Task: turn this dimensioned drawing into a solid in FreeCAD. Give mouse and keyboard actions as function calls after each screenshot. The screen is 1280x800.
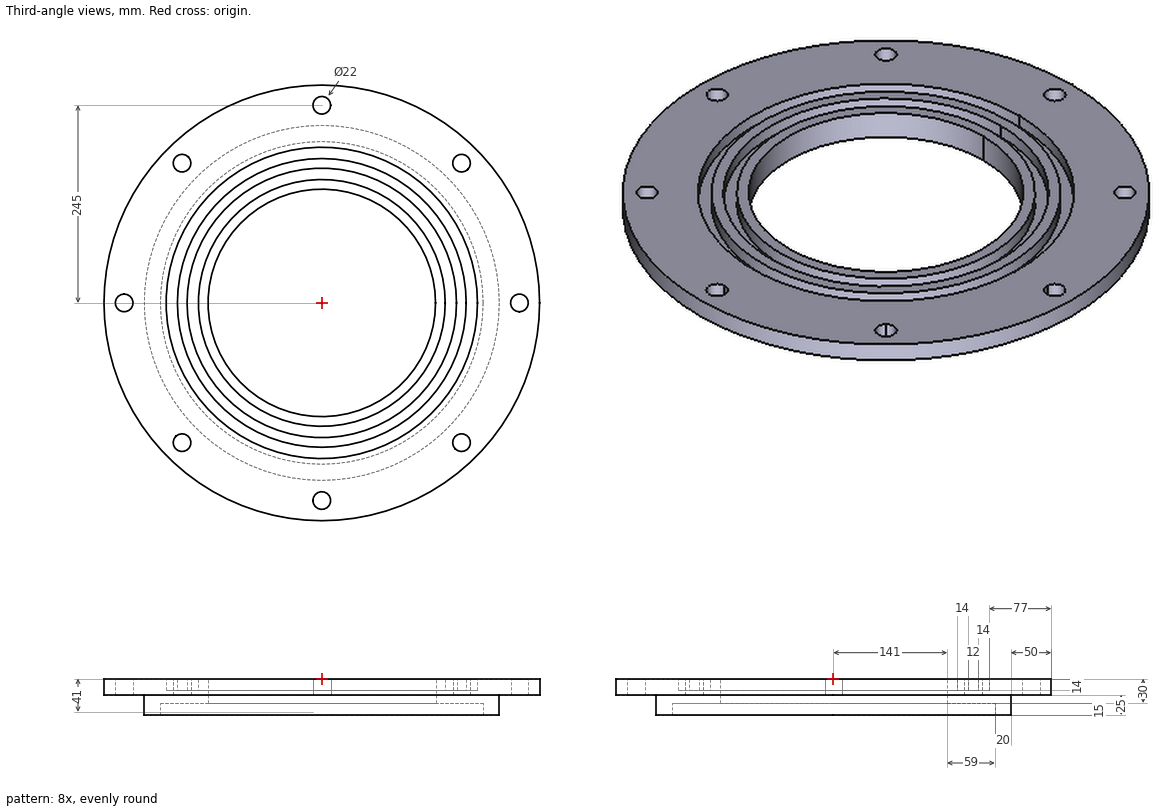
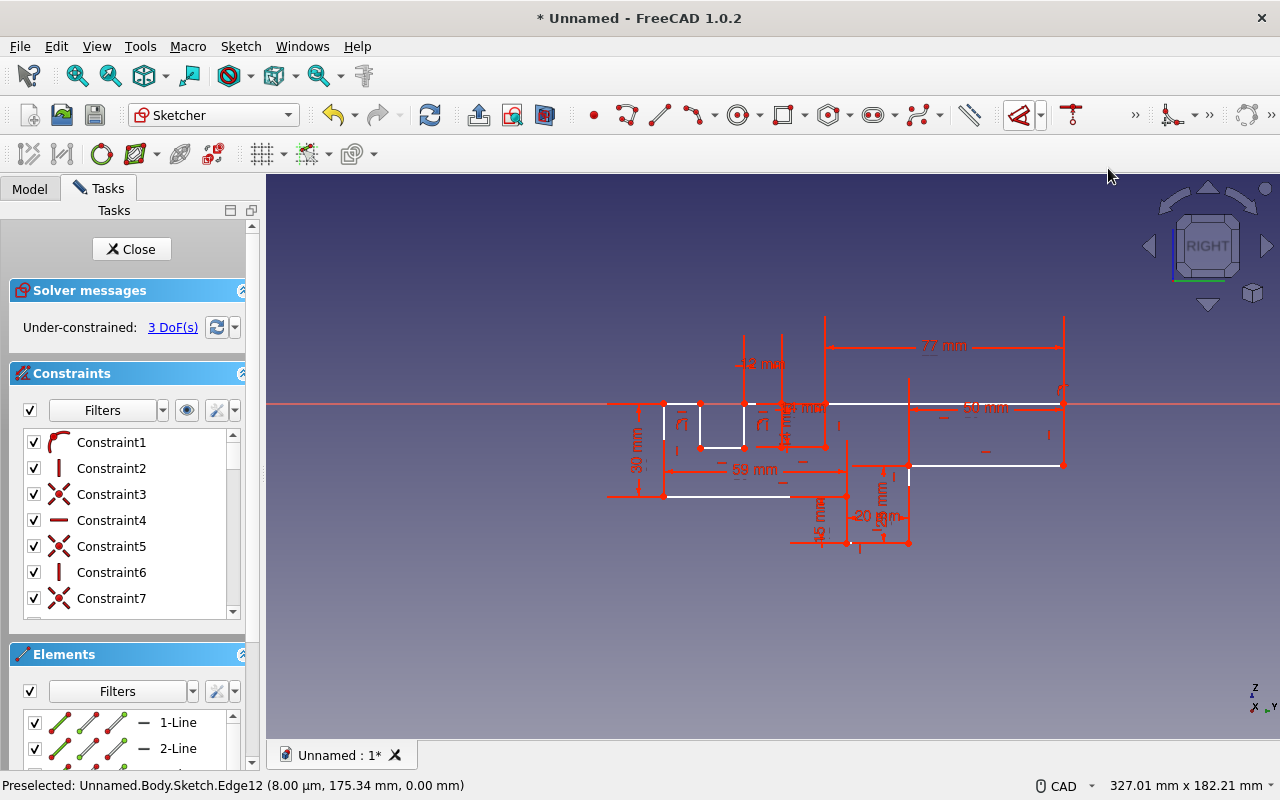
click(744, 417)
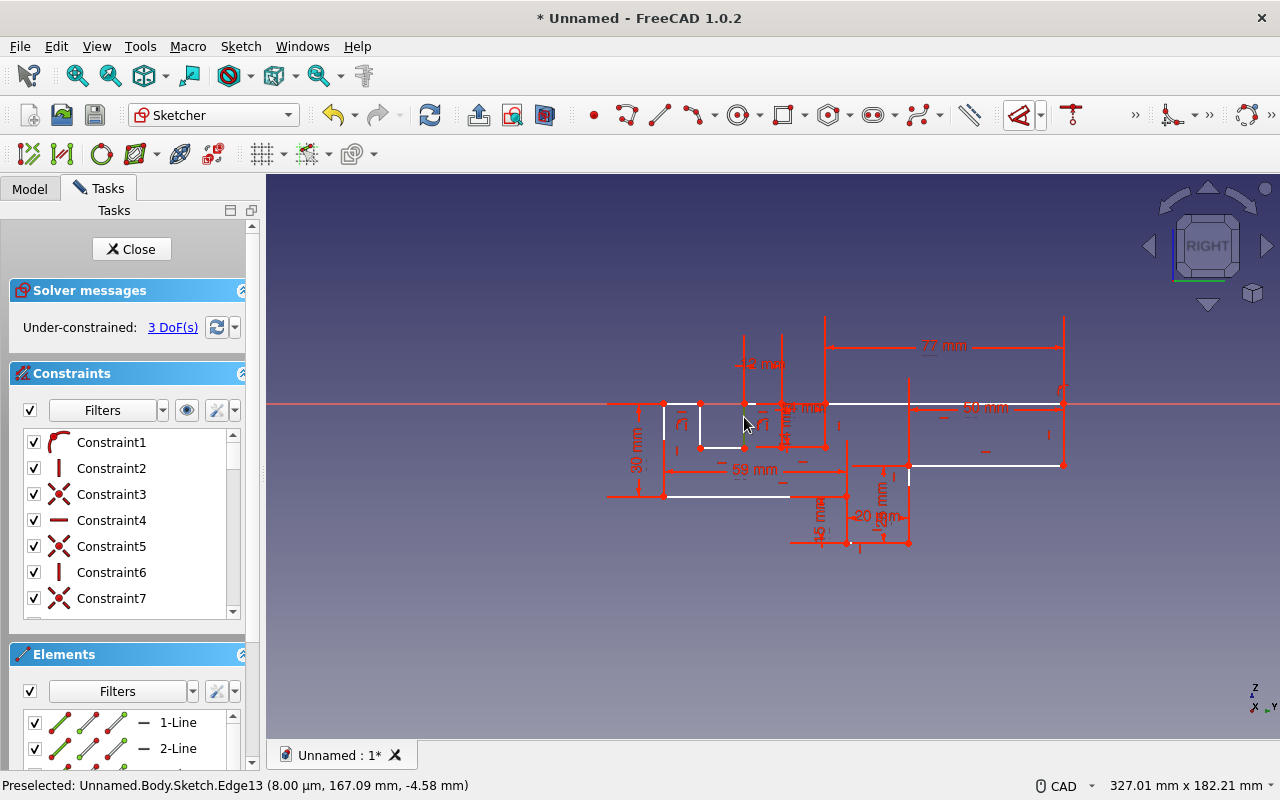
key(i)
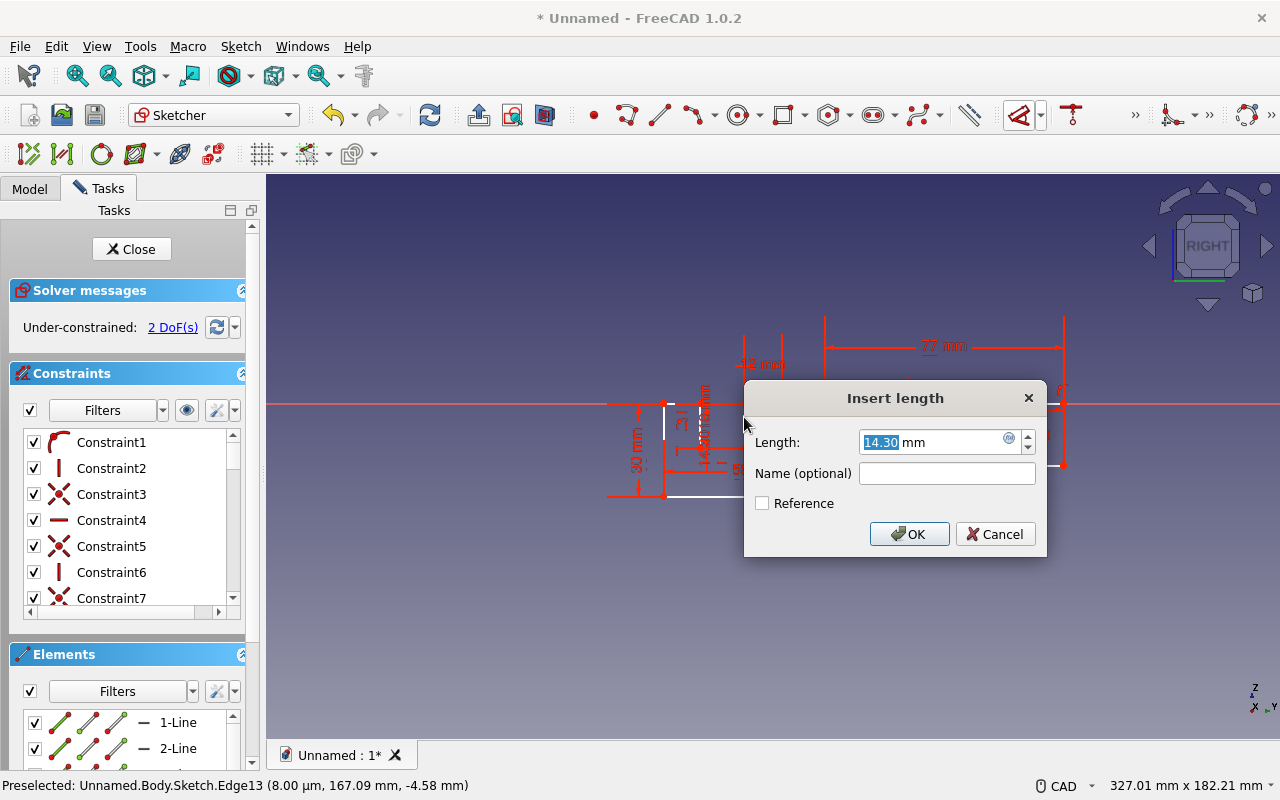
text(14)
key(Return)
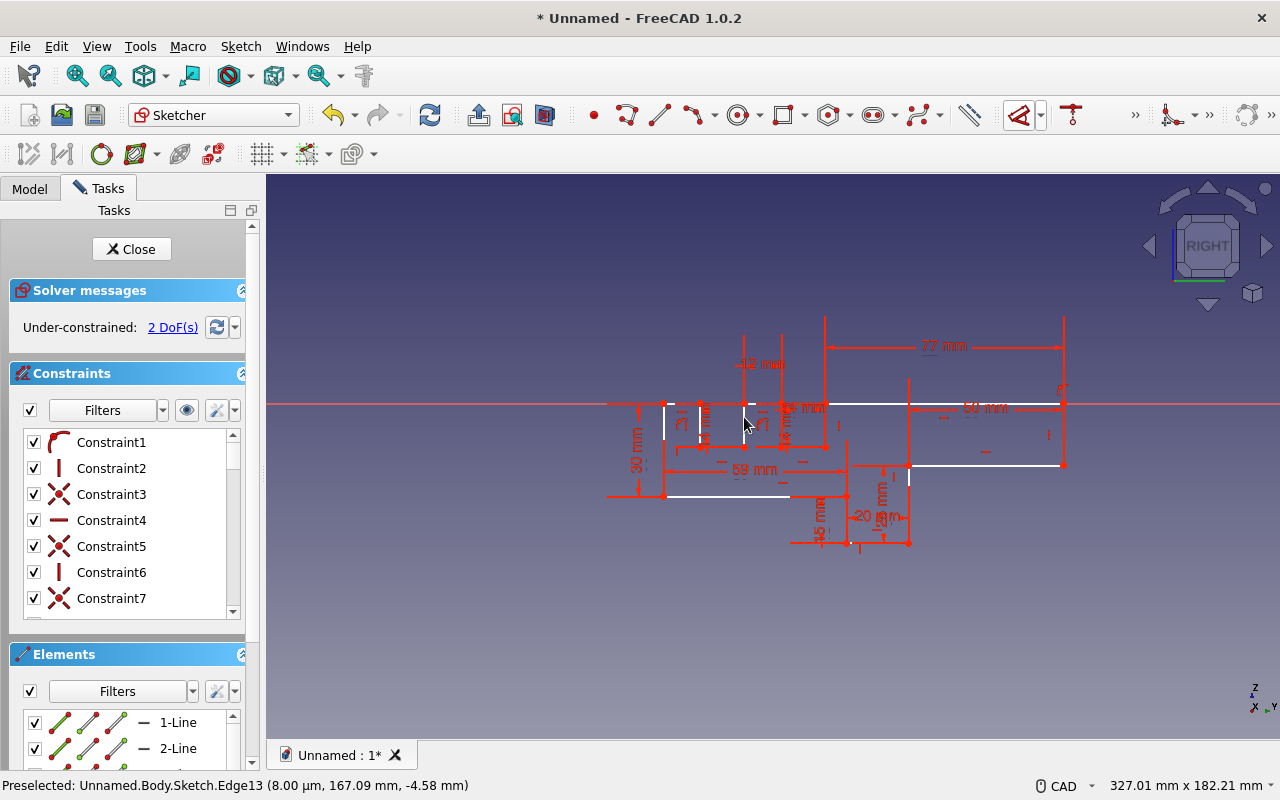
click(731, 447)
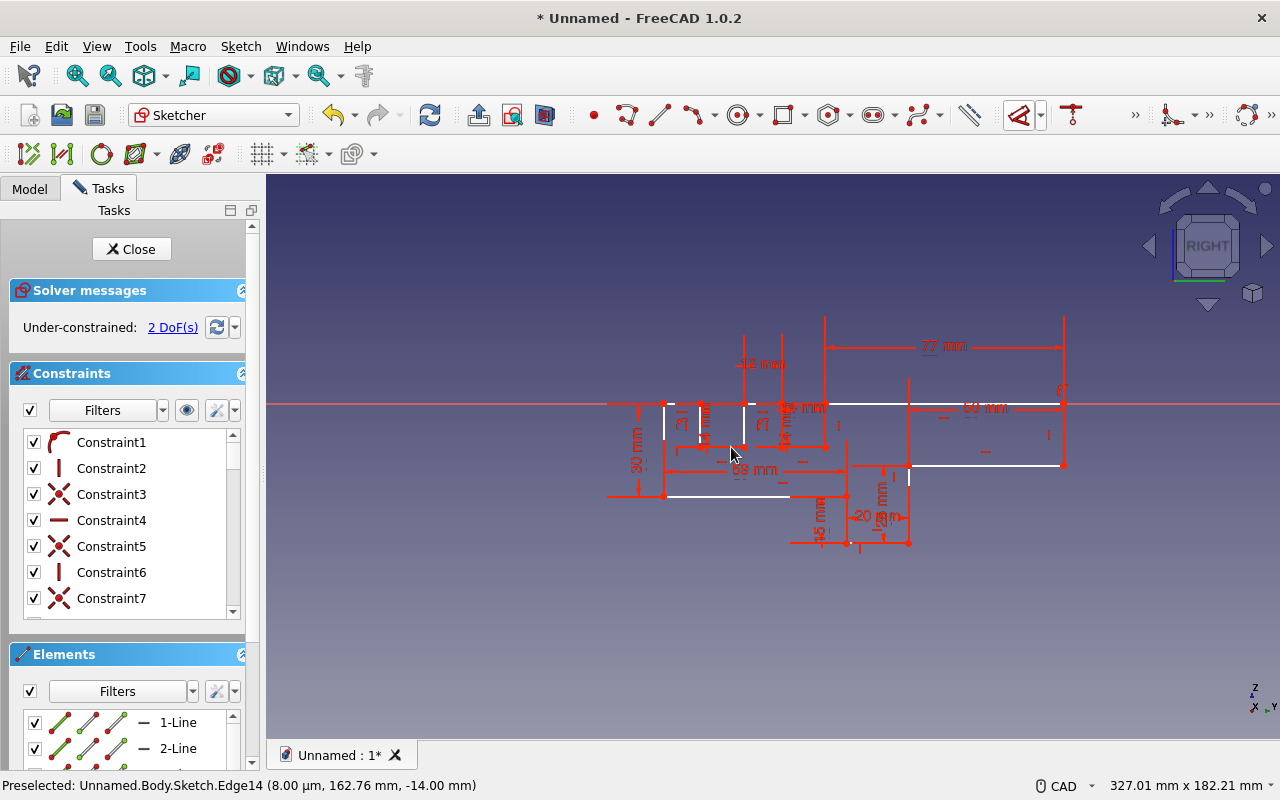
click(1040, 116)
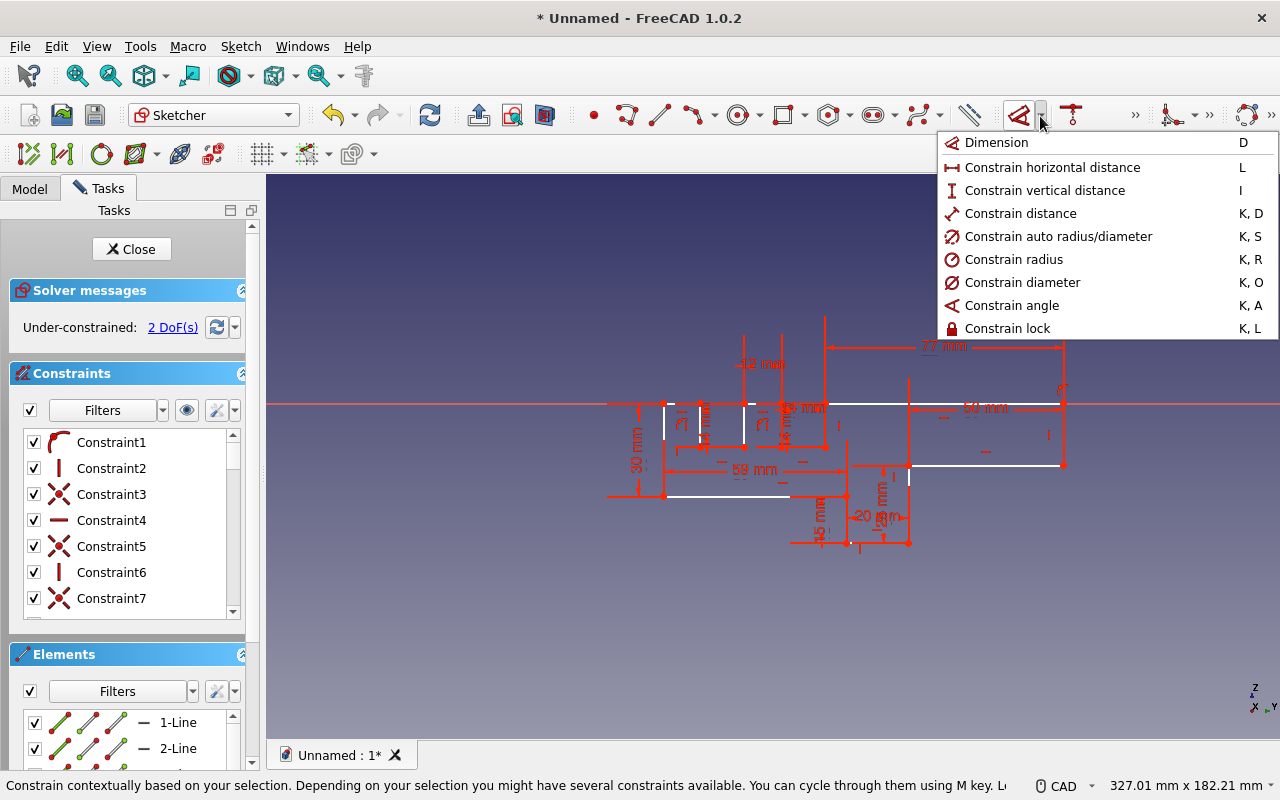
click(1108, 168)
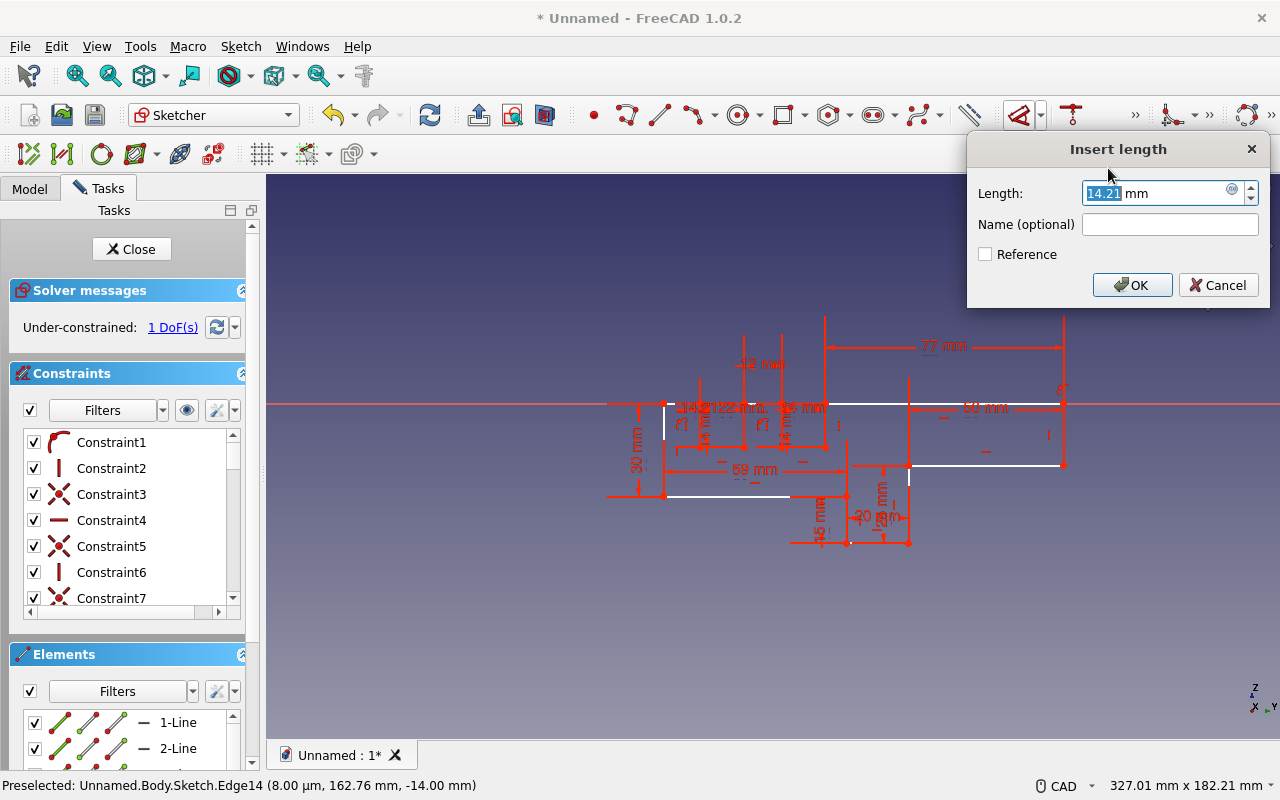
text(14)
key(Return)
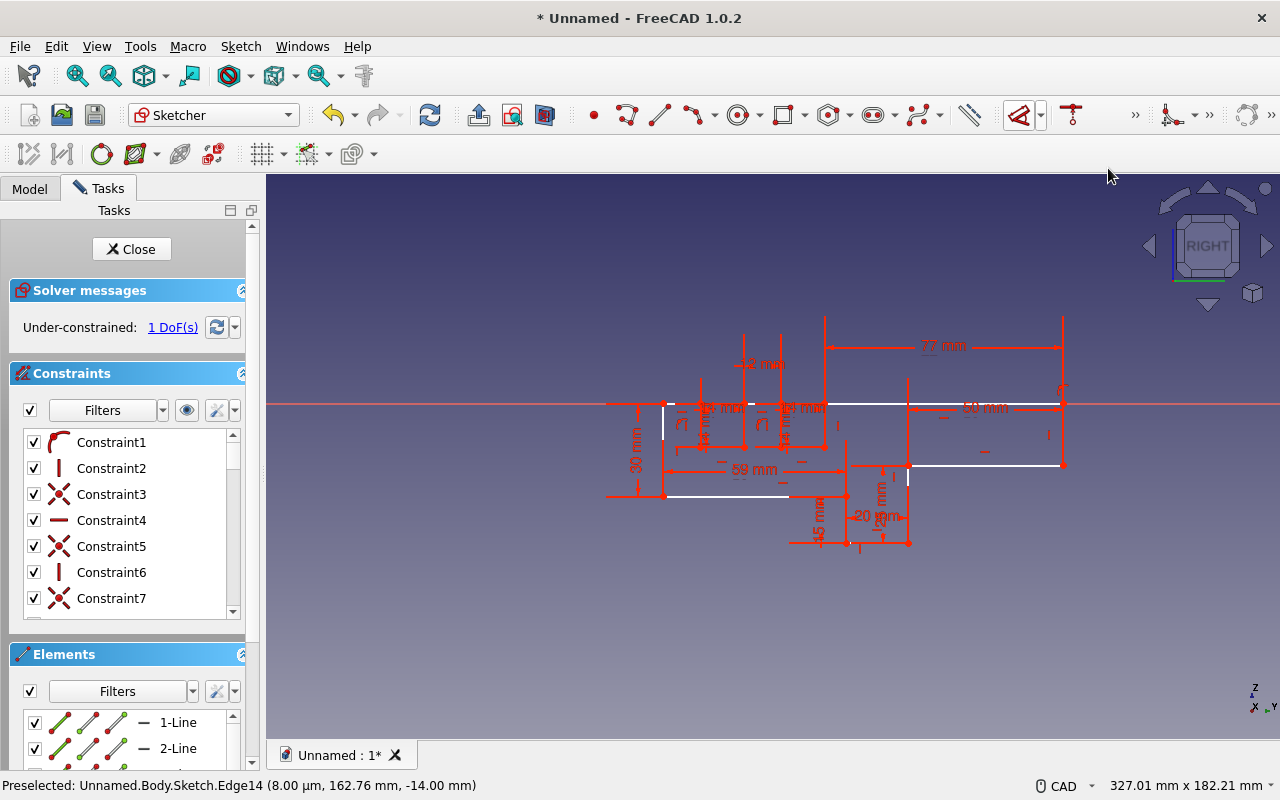
click(663, 404)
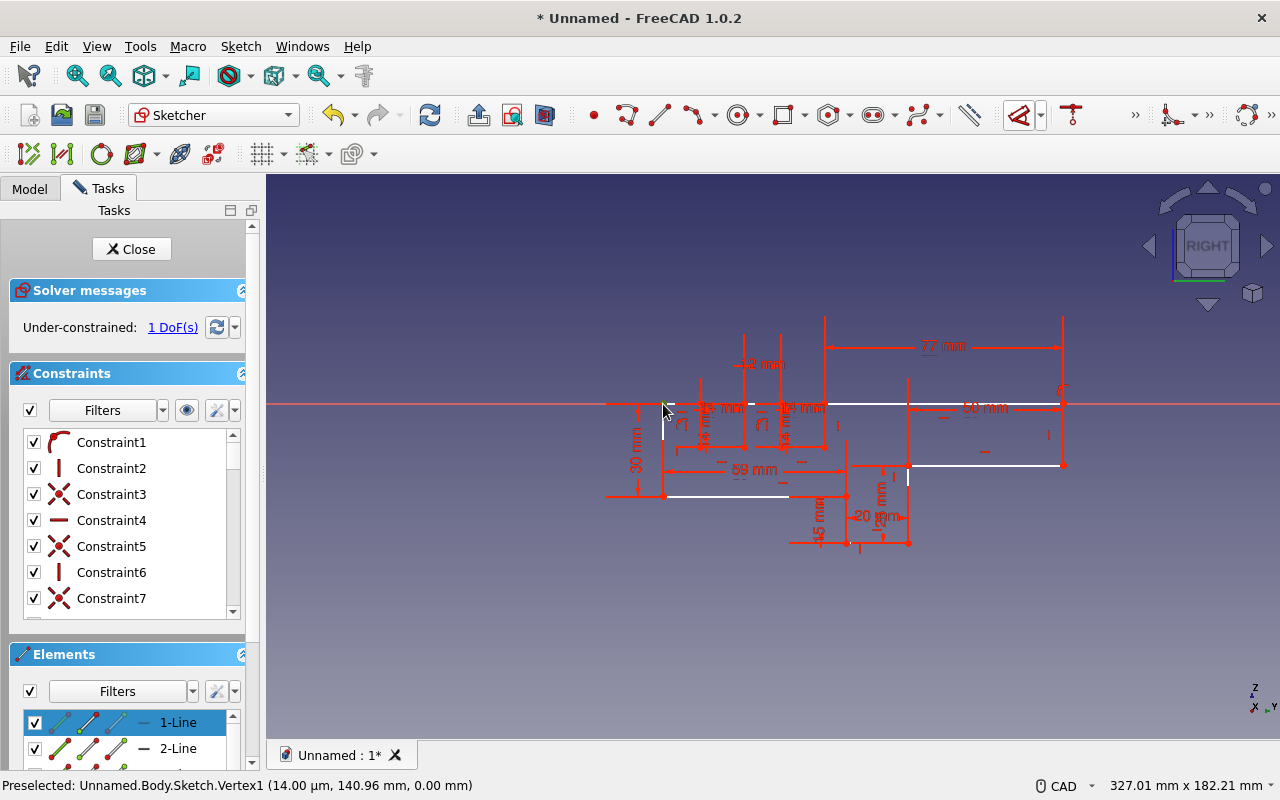
click(1040, 116)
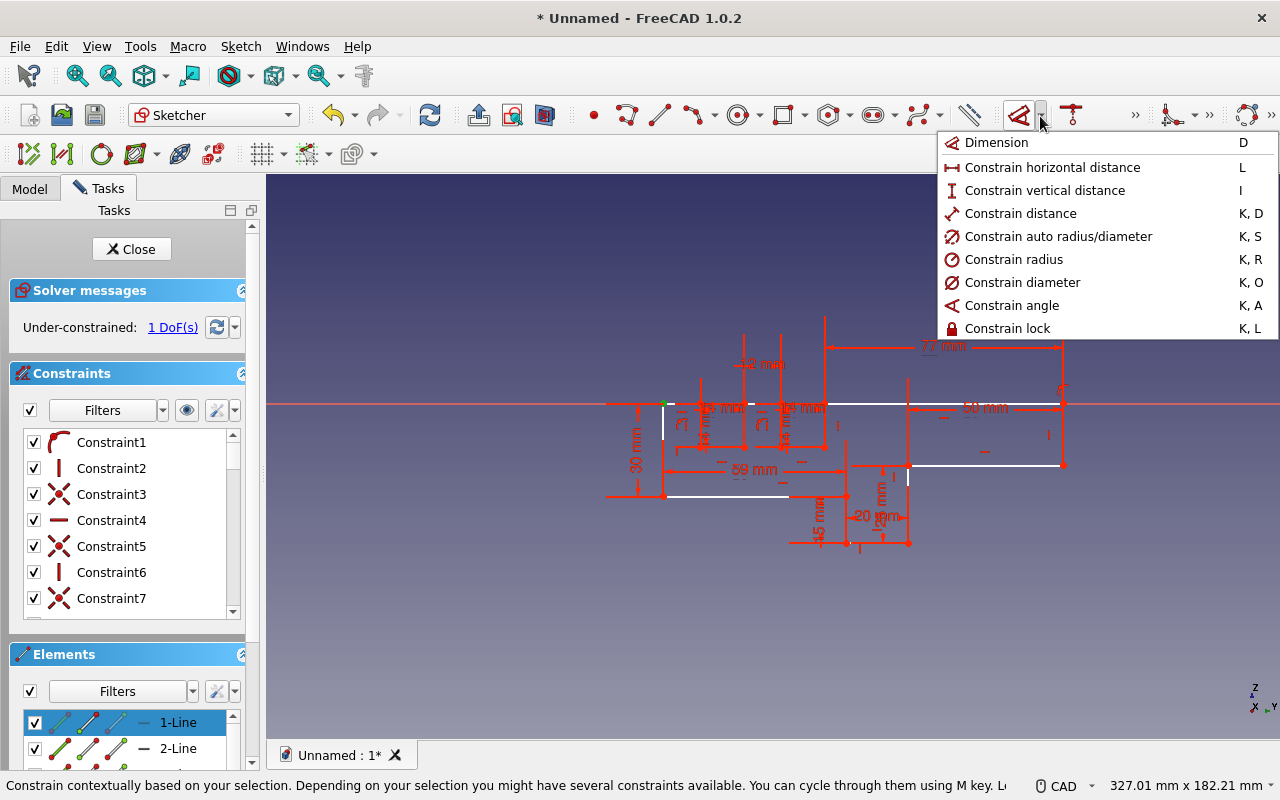
click(1108, 168)